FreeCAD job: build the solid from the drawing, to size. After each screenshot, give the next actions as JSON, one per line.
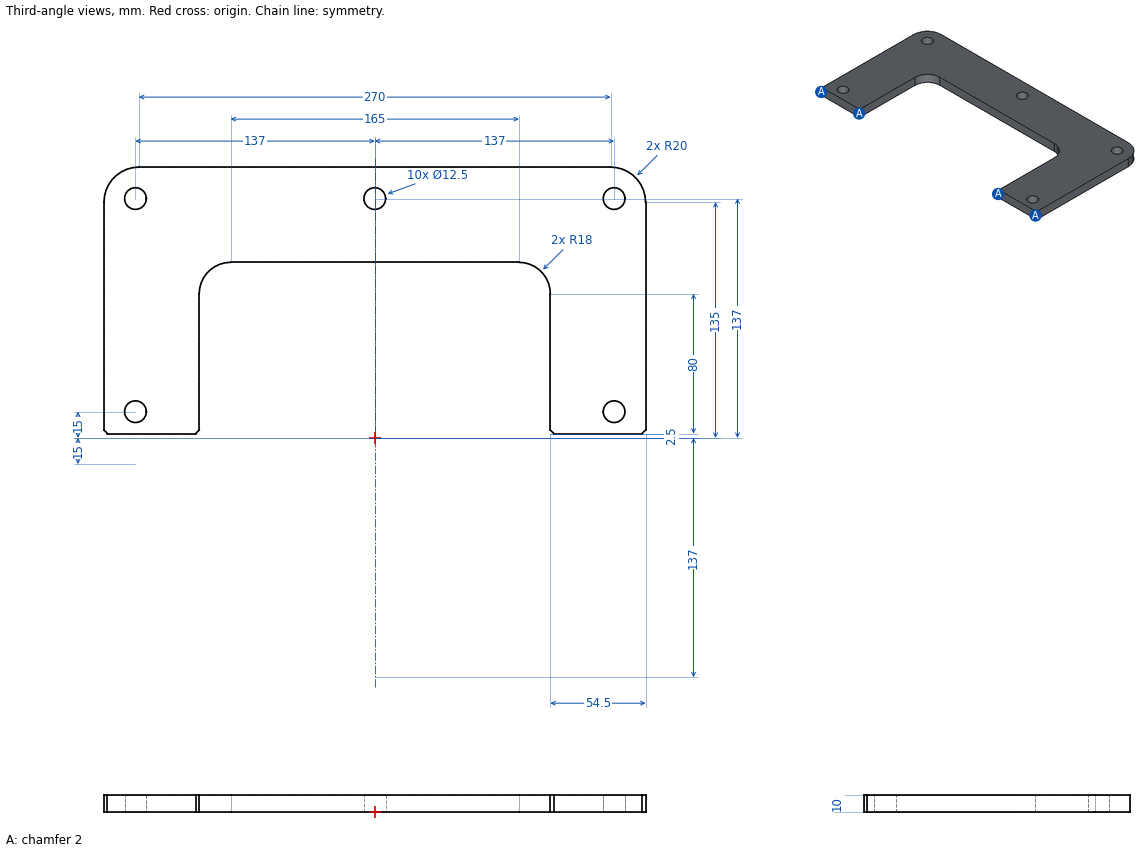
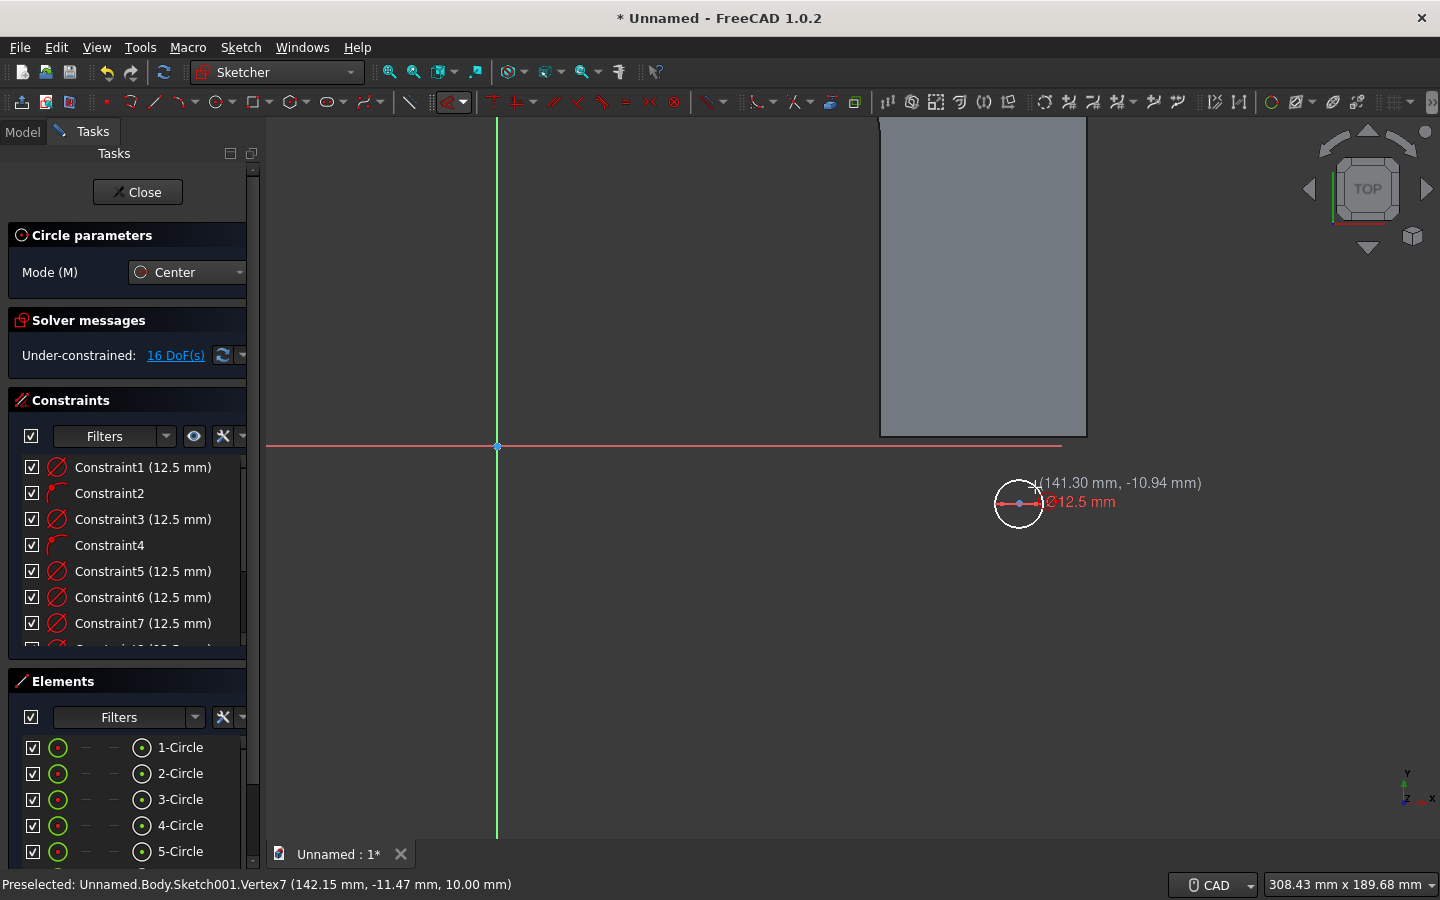
{"action": "left_click", "coordinate": [1019, 389]}
{"action": "mouse_move", "coordinate": [1035, 372]}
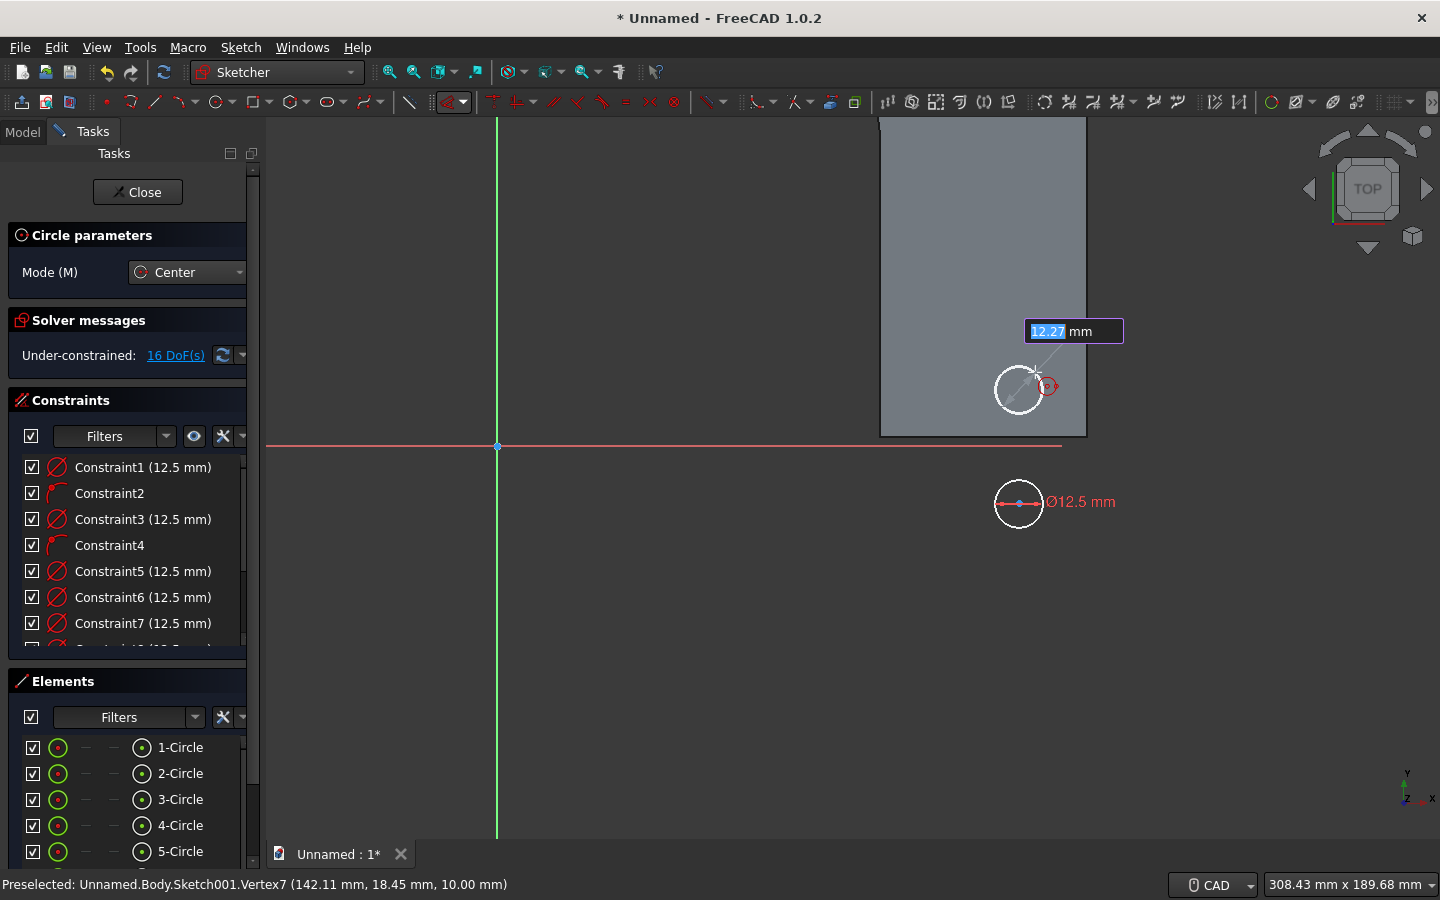
{"action": "type", "text": "12.5"}
{"action": "key", "text": "Return"}
{"action": "key", "text": "Escape"}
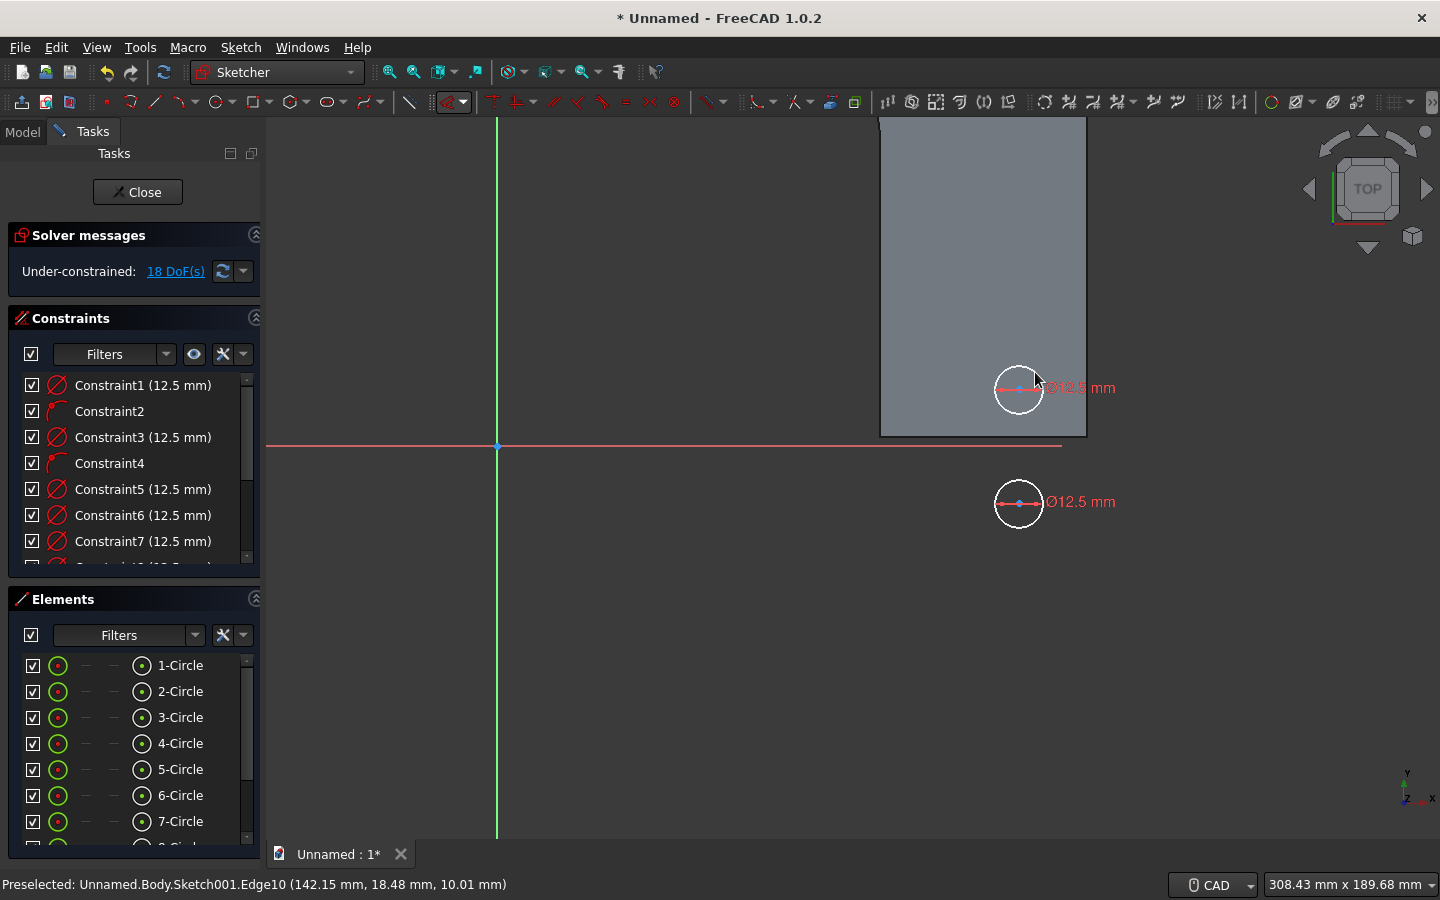
{"action": "scroll", "coordinate": [1019, 504], "scroll_direction": "down", "scroll_amount": 4}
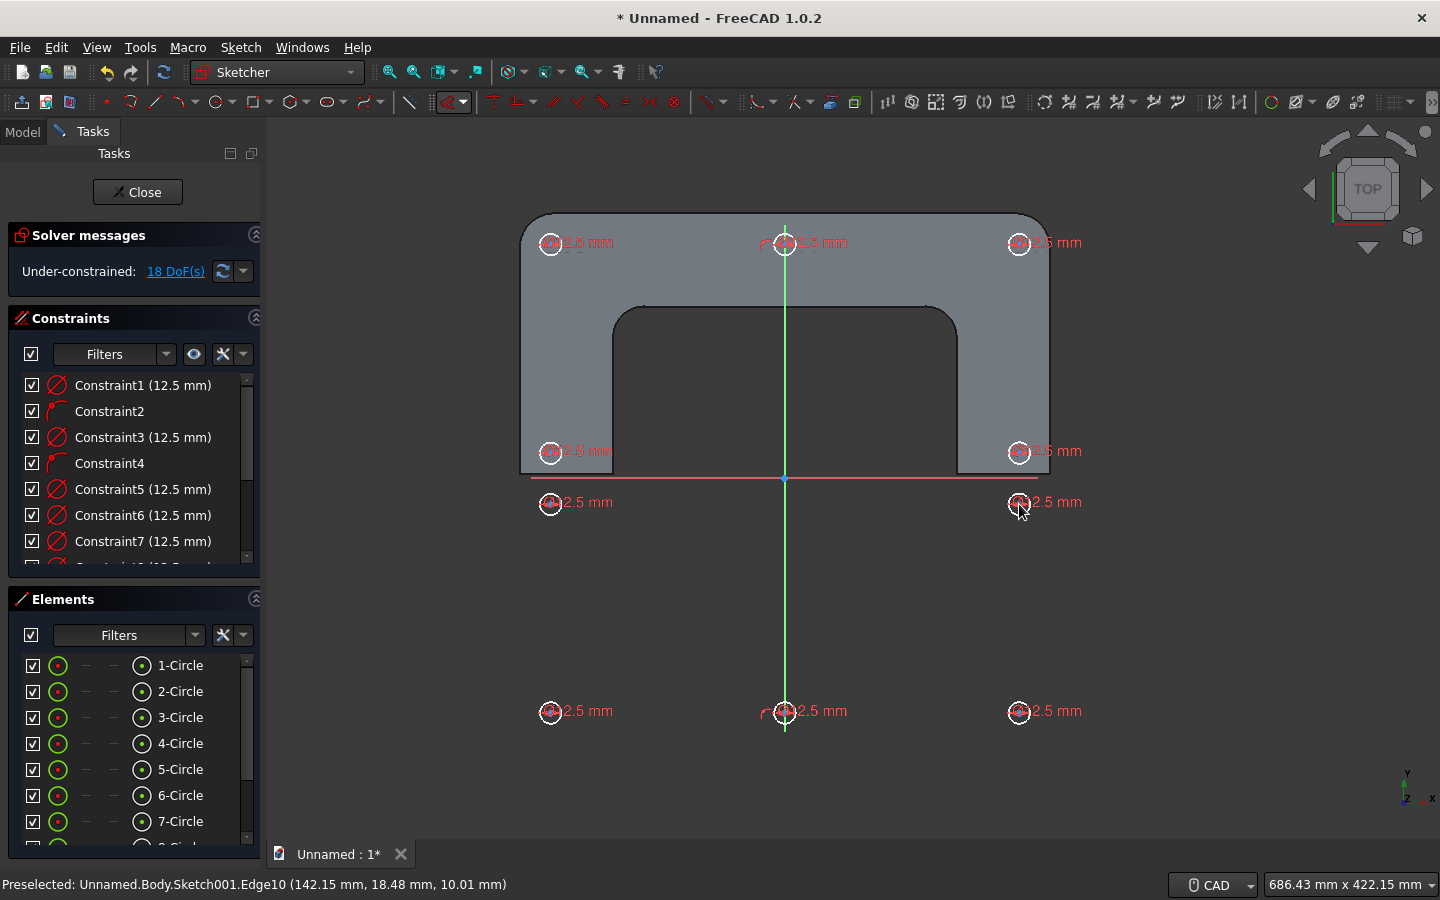
{"action": "left_click", "coordinate": [785, 245]}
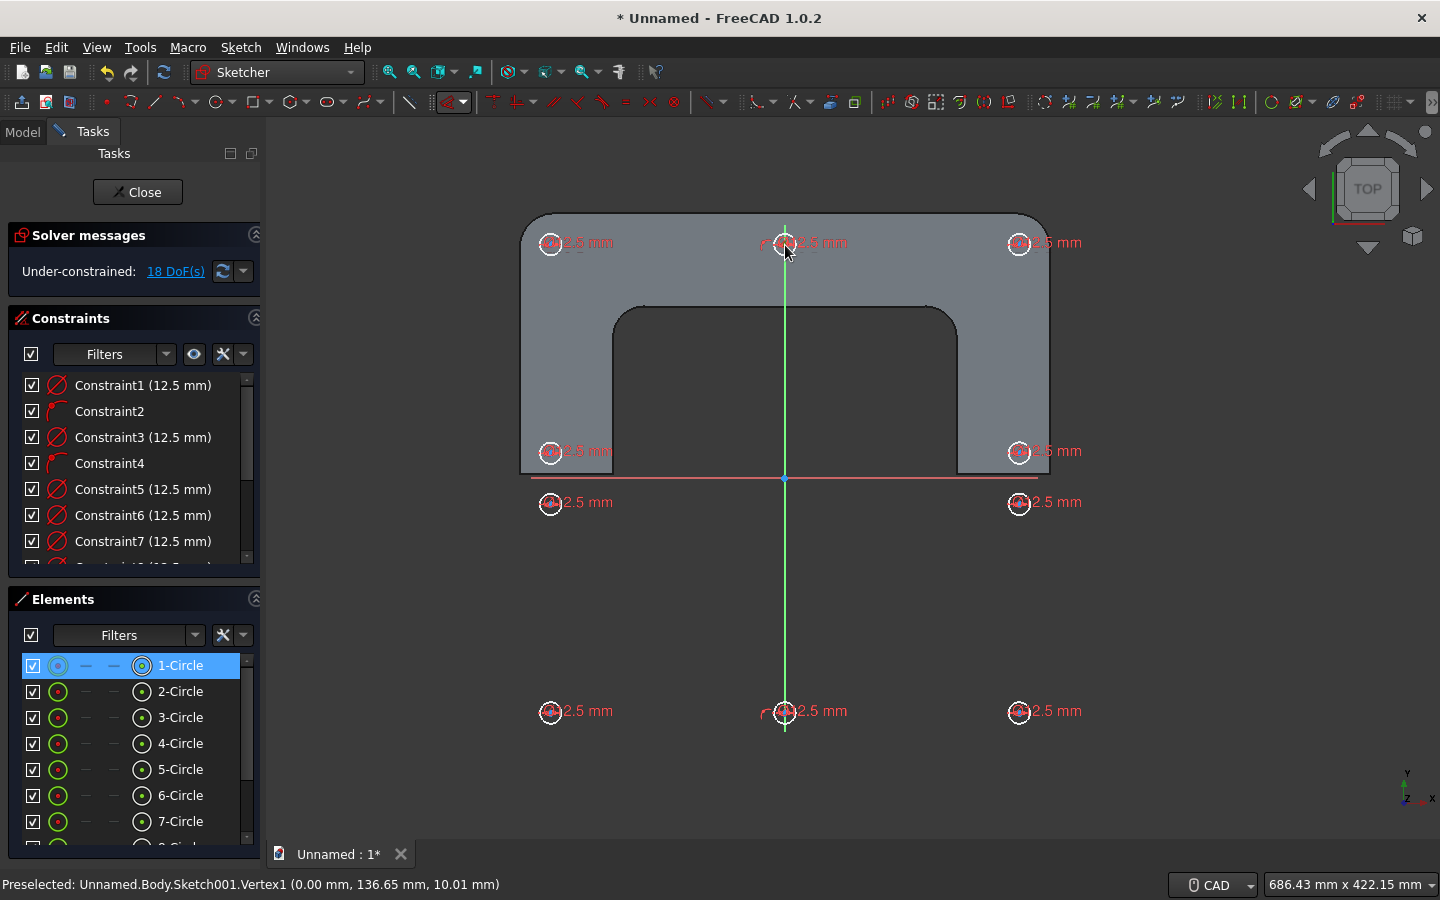
{"action": "left_click", "coordinate": [551, 245]}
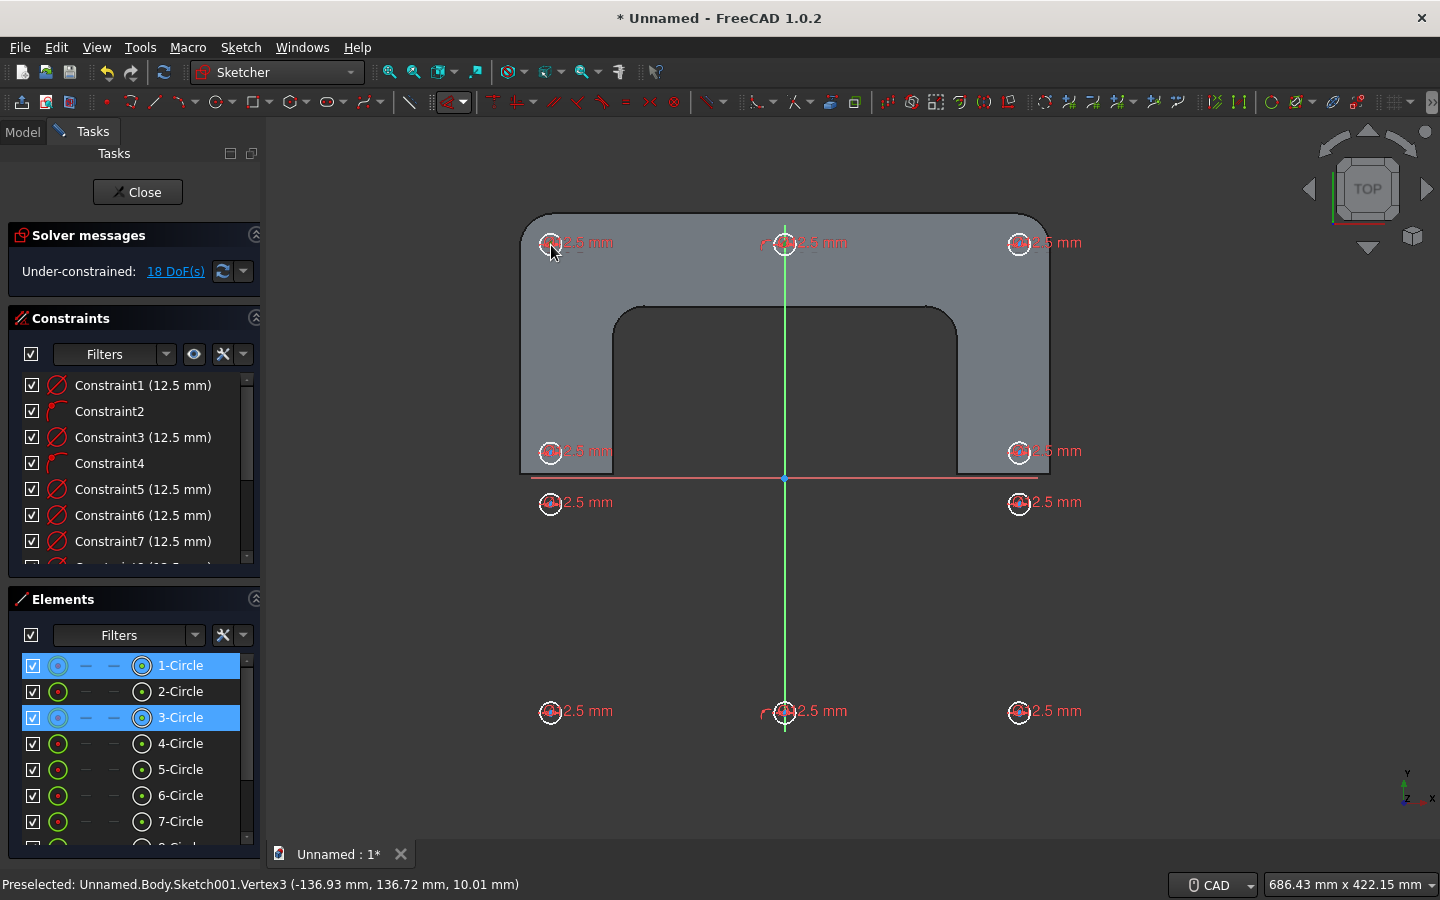
{"action": "key", "text": "h"}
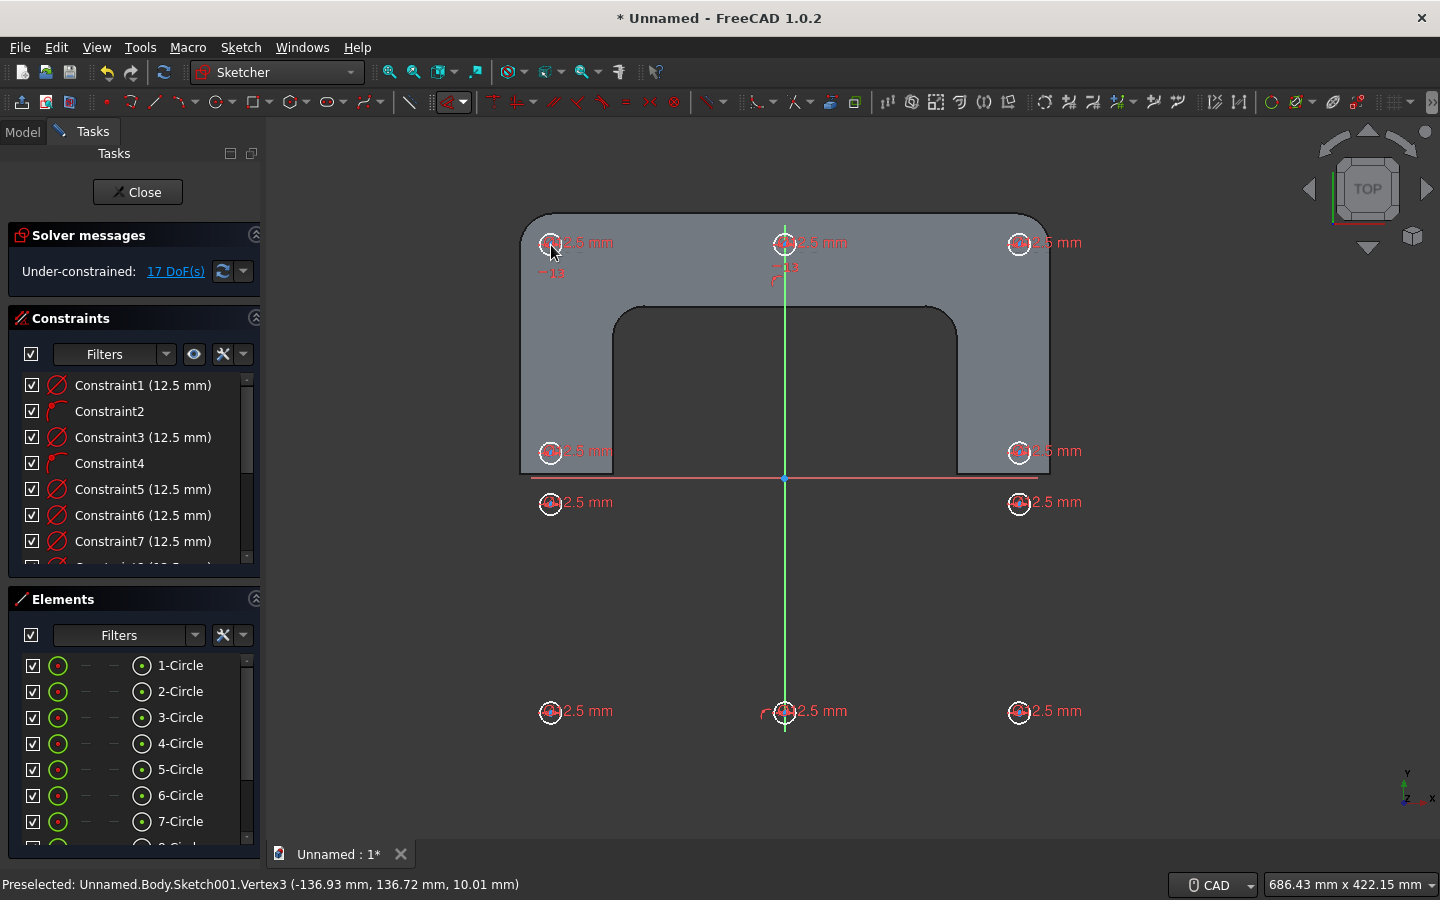
{"action": "left_click", "coordinate": [785, 245]}